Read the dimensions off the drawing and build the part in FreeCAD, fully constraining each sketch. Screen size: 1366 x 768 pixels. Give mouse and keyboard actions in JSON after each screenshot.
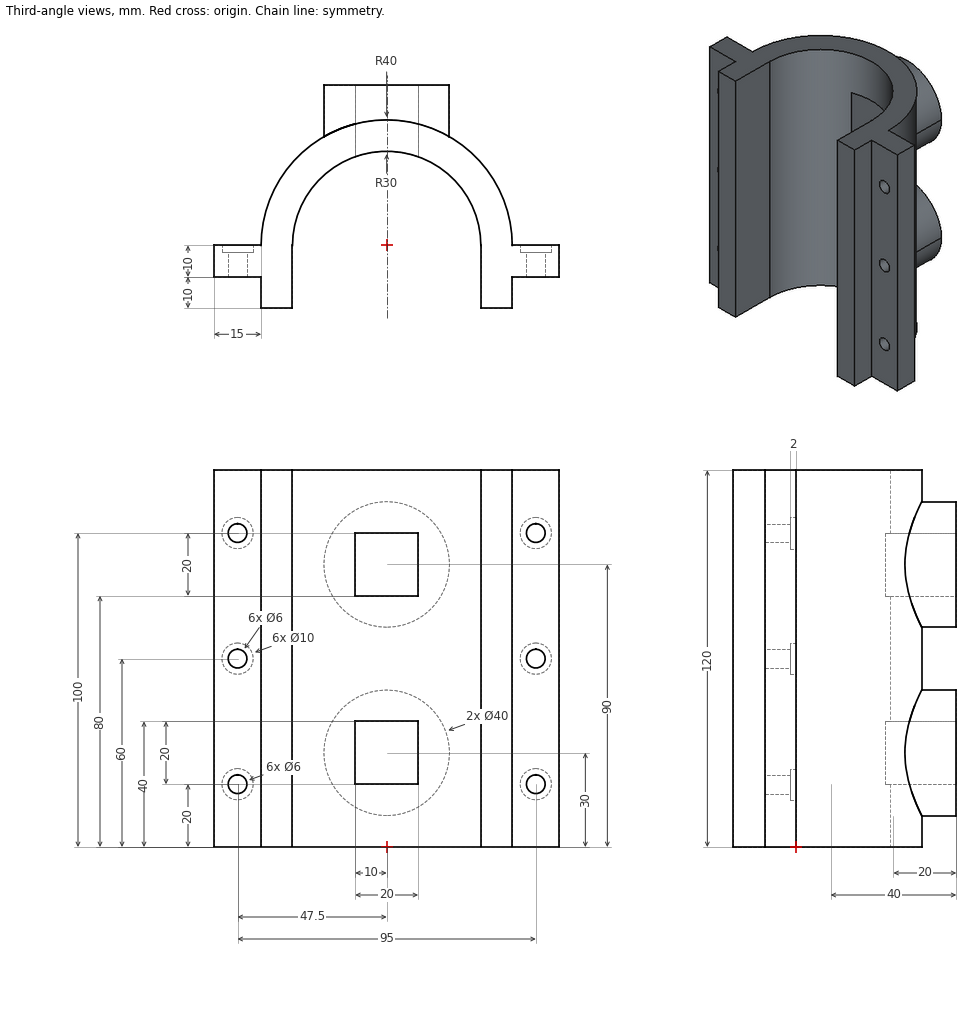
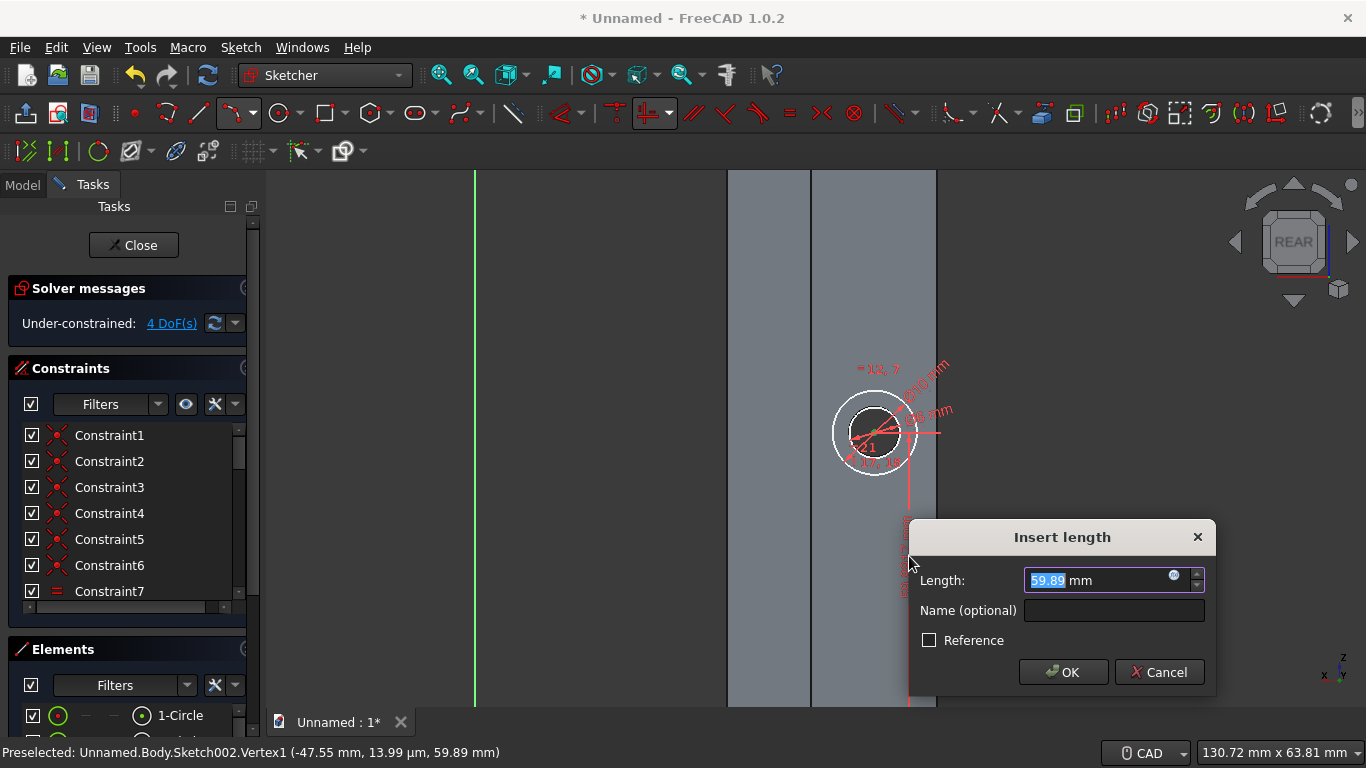
{"action": "type", "text": "60"}
{"action": "key", "text": "Return"}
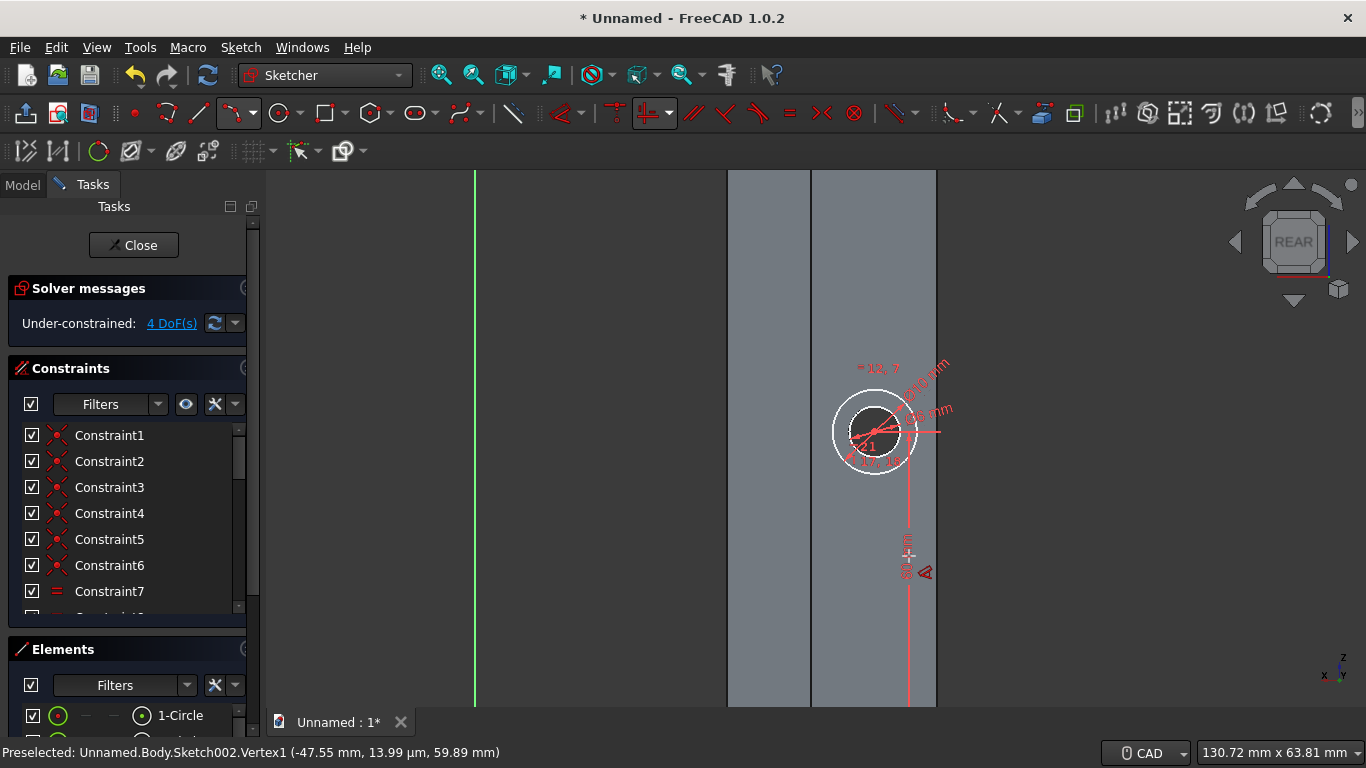
{"action": "scroll", "coordinate": [906, 406], "scroll_direction": "down", "scroll_amount": 5}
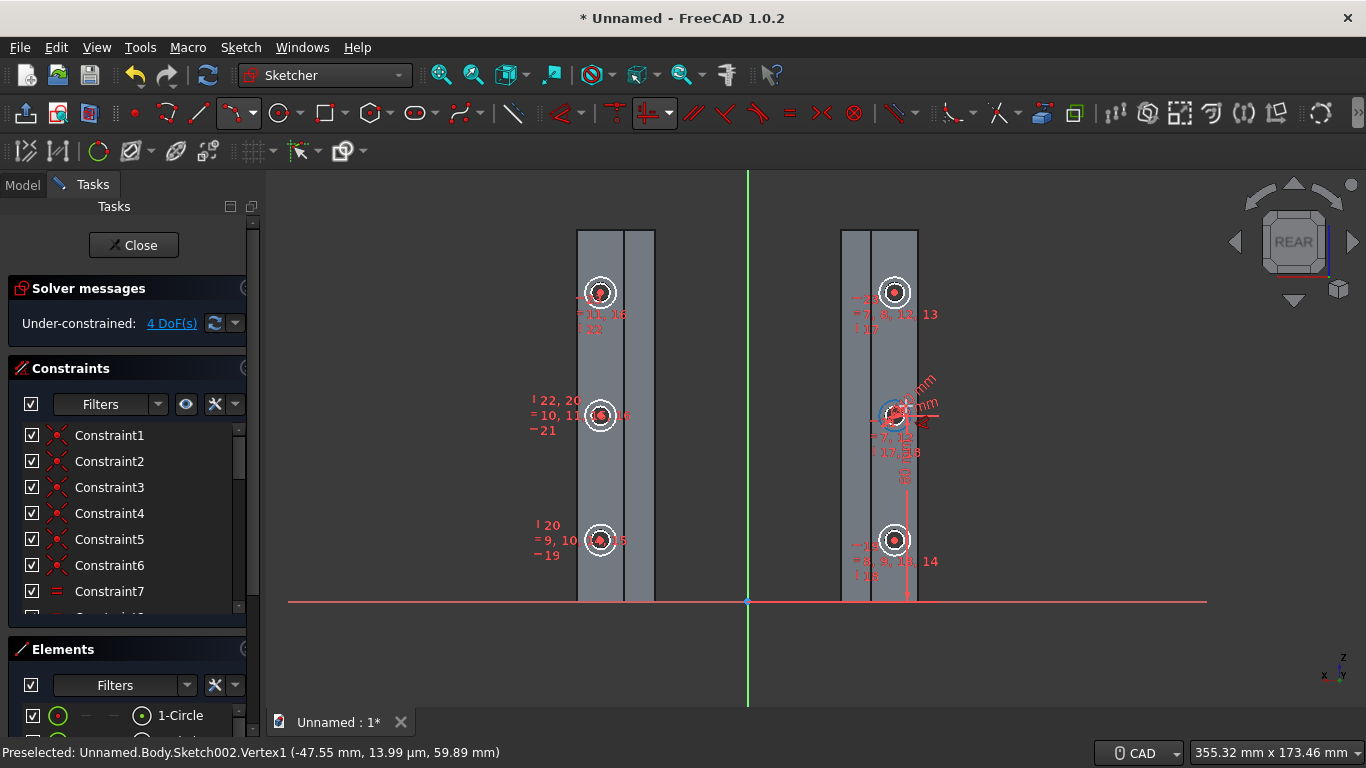
{"action": "left_click", "coordinate": [895, 540]}
{"action": "left_click", "coordinate": [929, 571]}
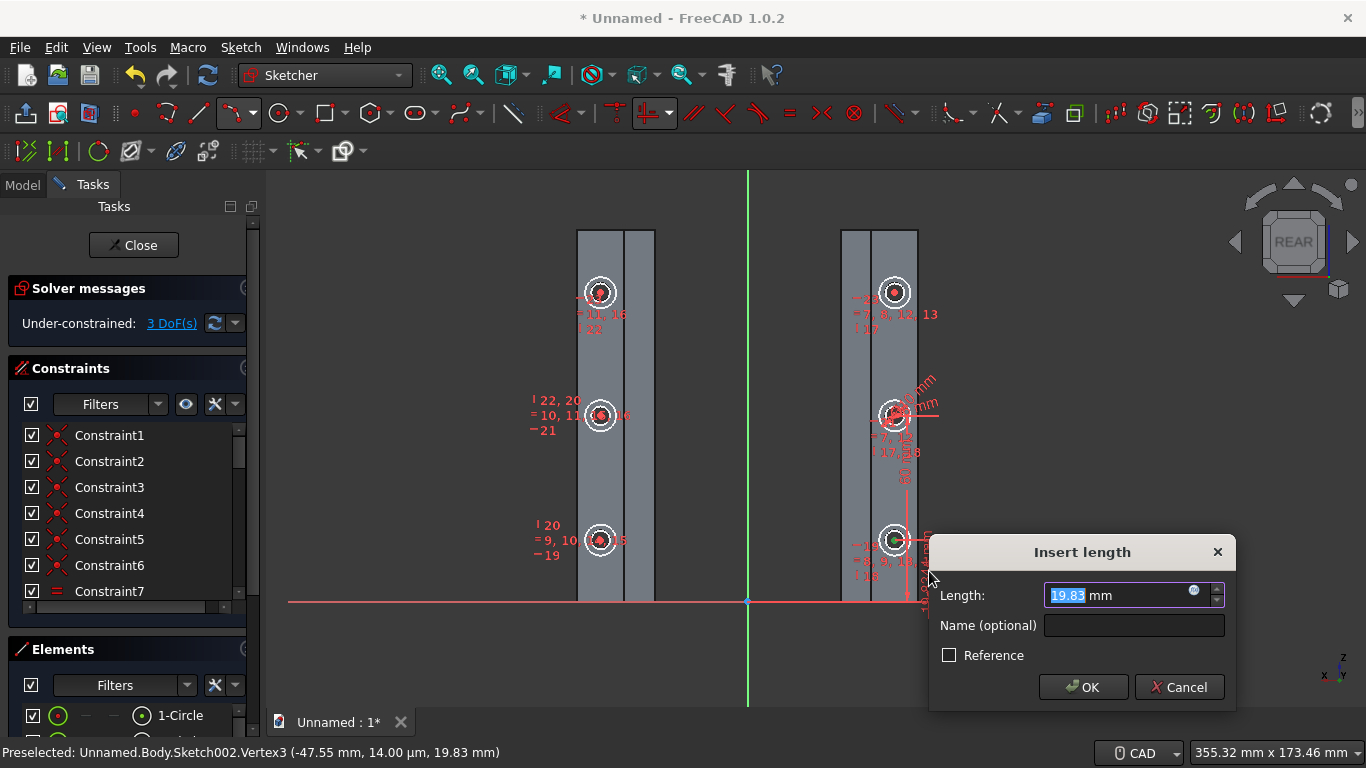
{"action": "type", "text": "20"}
{"action": "key", "text": "Return"}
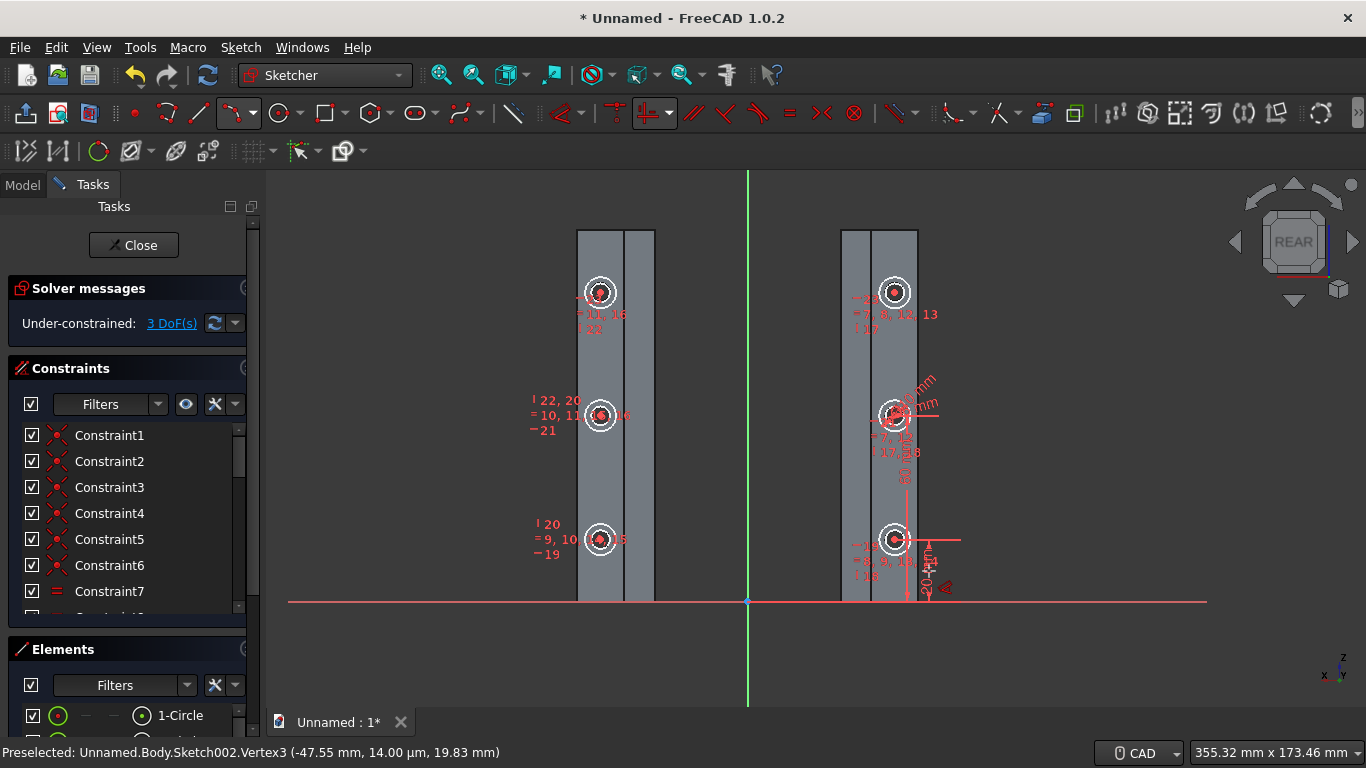
{"action": "left_click", "coordinate": [895, 293]}
{"action": "left_click", "coordinate": [929, 376]}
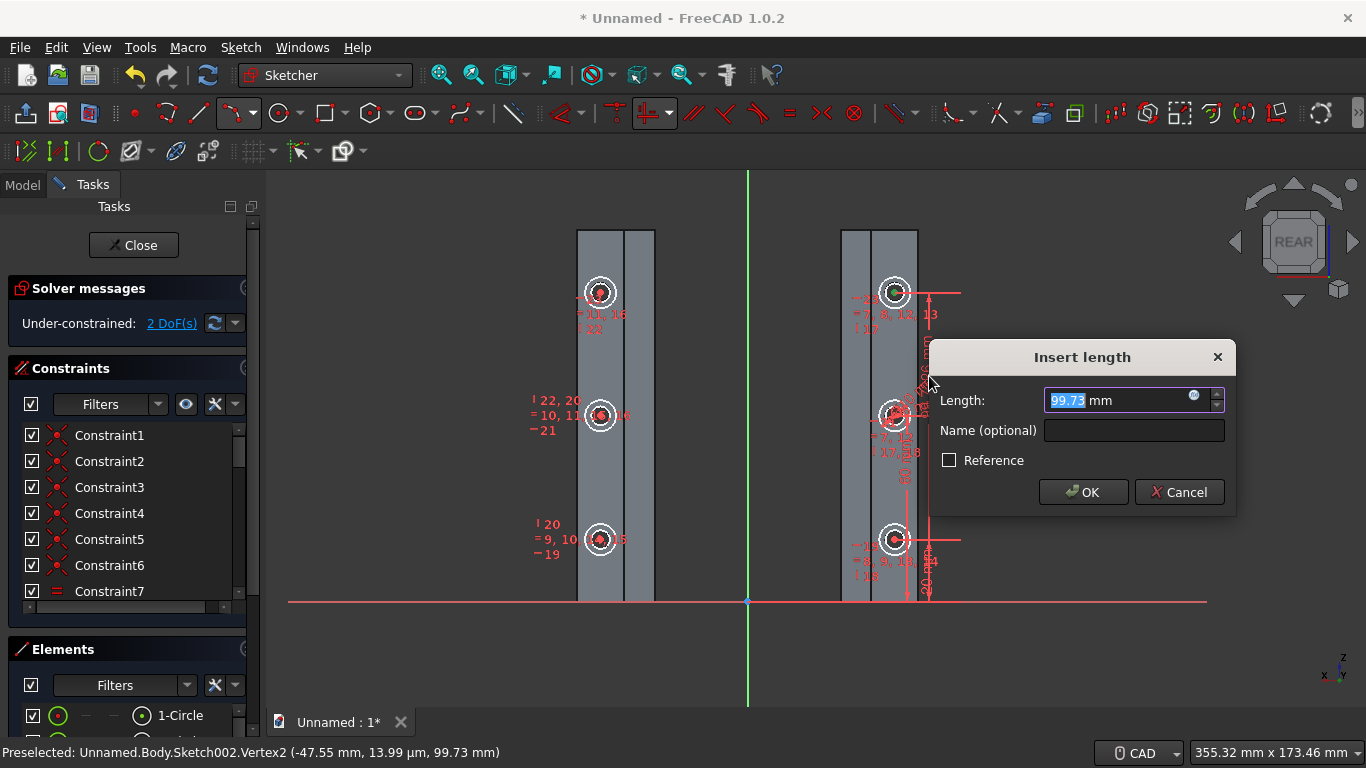
{"action": "type", "text": "100"}
{"action": "key", "text": "Return"}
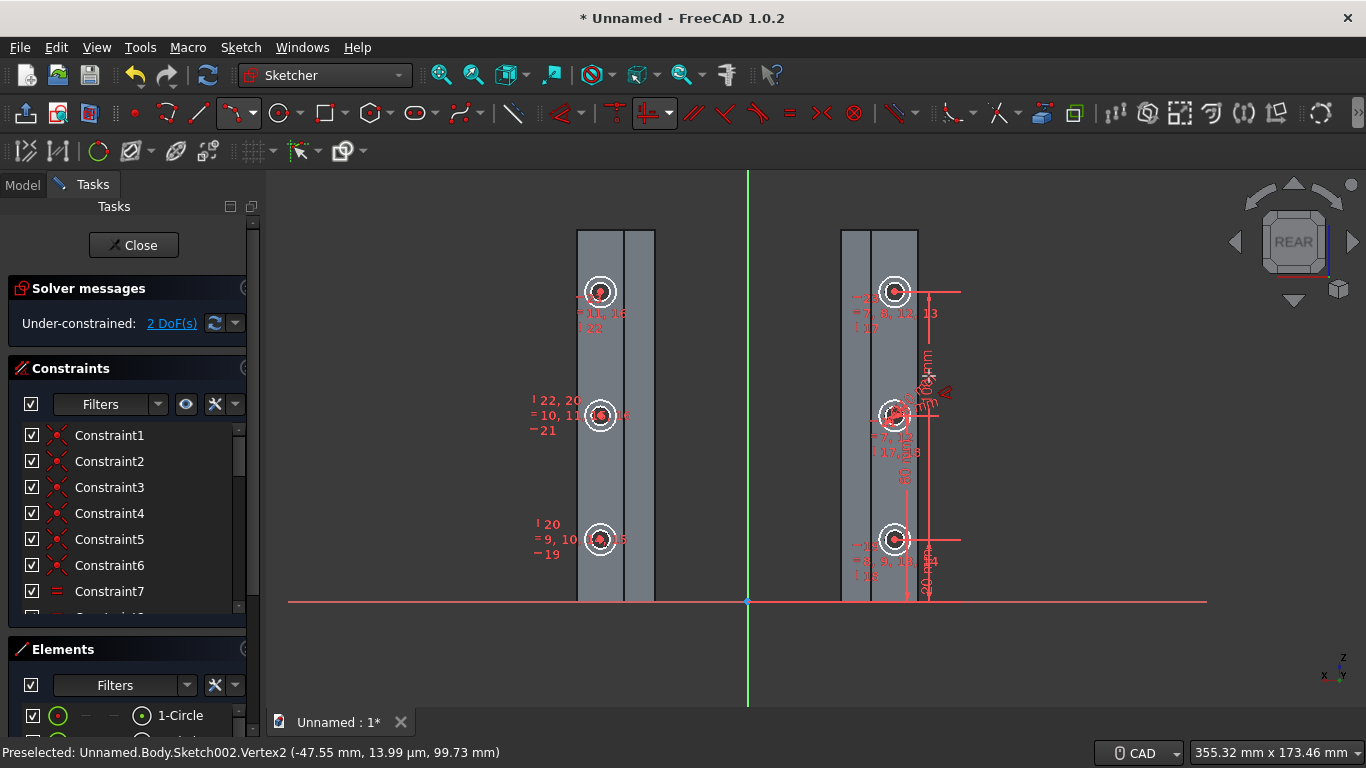
{"action": "left_click", "coordinate": [895, 540]}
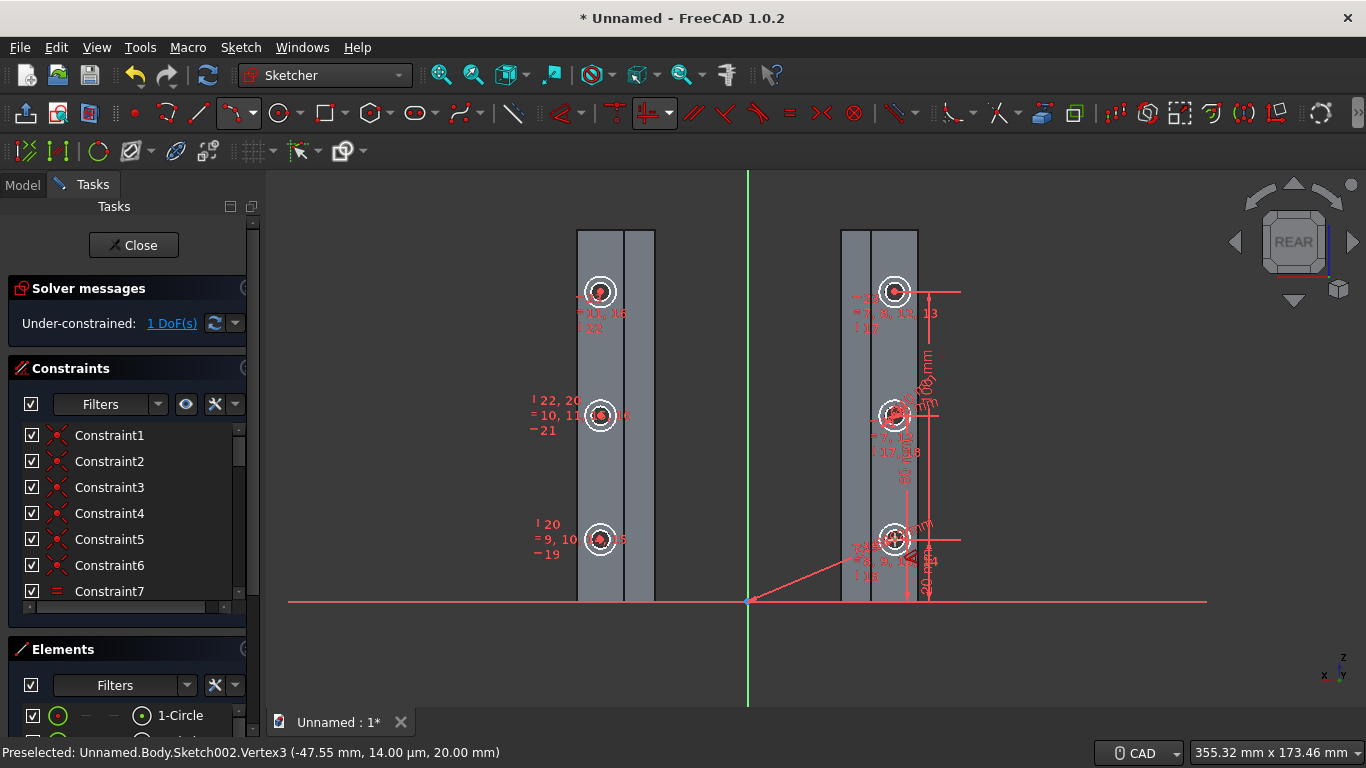
{"action": "left_click", "coordinate": [601, 540]}
{"action": "left_click", "coordinate": [680, 574]}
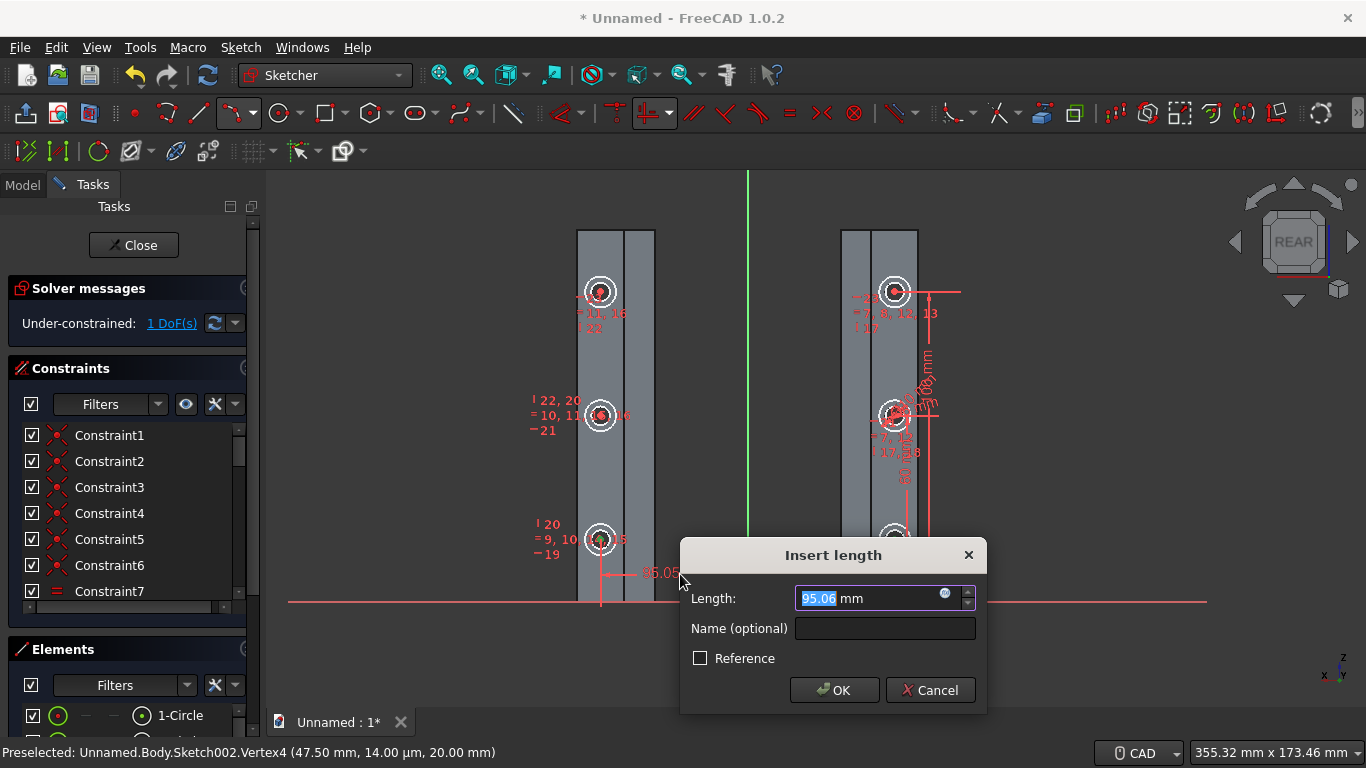
{"action": "type", "text": "95"}
{"action": "key", "text": "Return"}